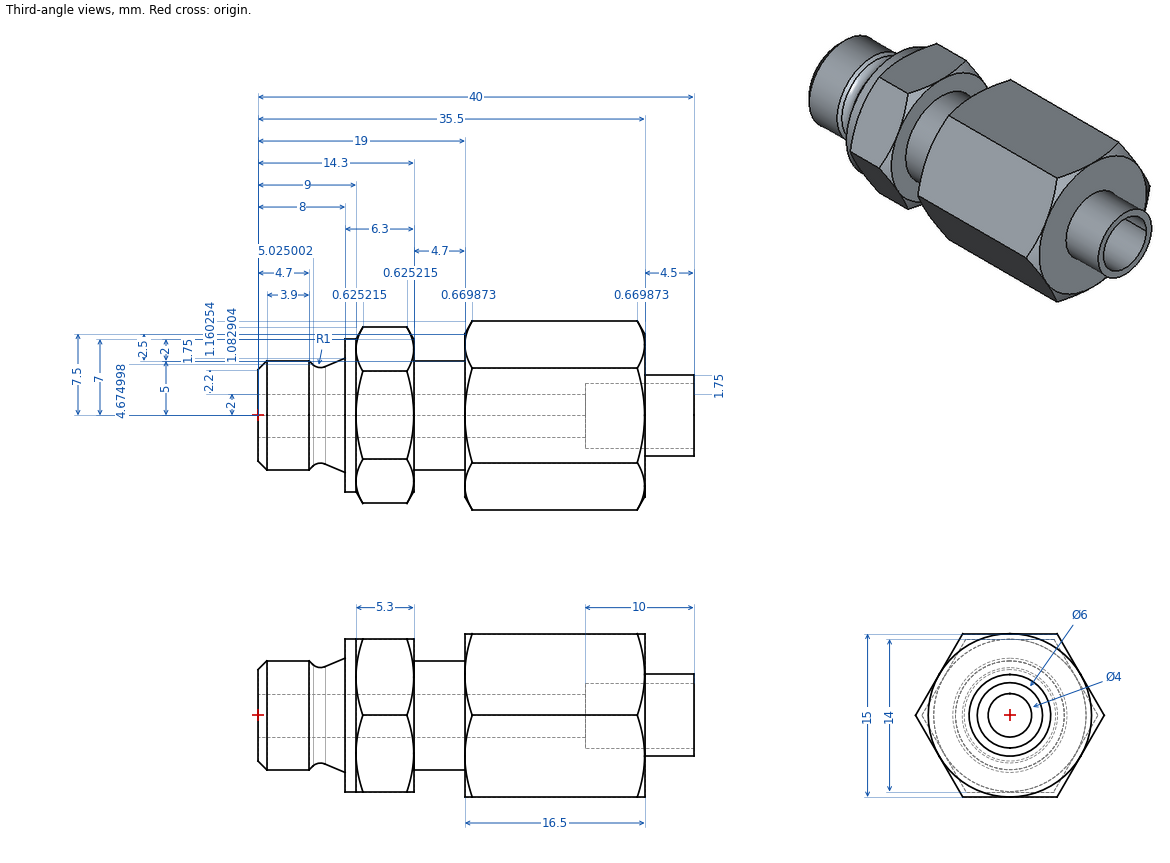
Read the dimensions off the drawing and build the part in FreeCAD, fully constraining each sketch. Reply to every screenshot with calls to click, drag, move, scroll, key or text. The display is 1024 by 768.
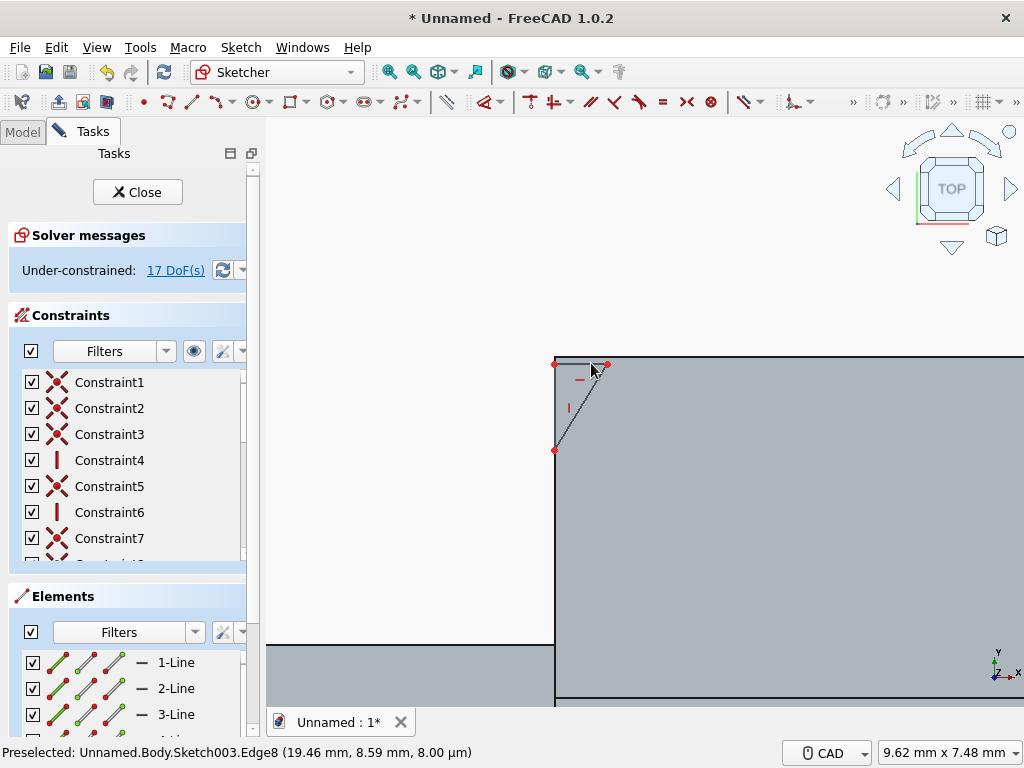
scroll(595, 367, down, 10)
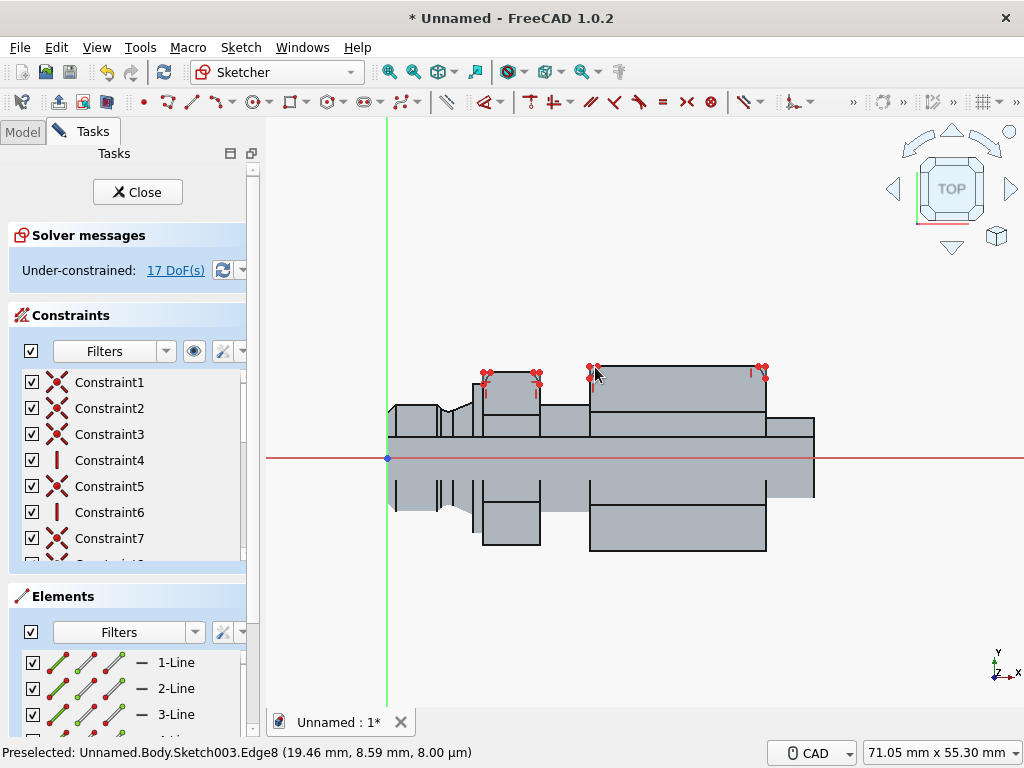
scroll(764, 366, up, 10)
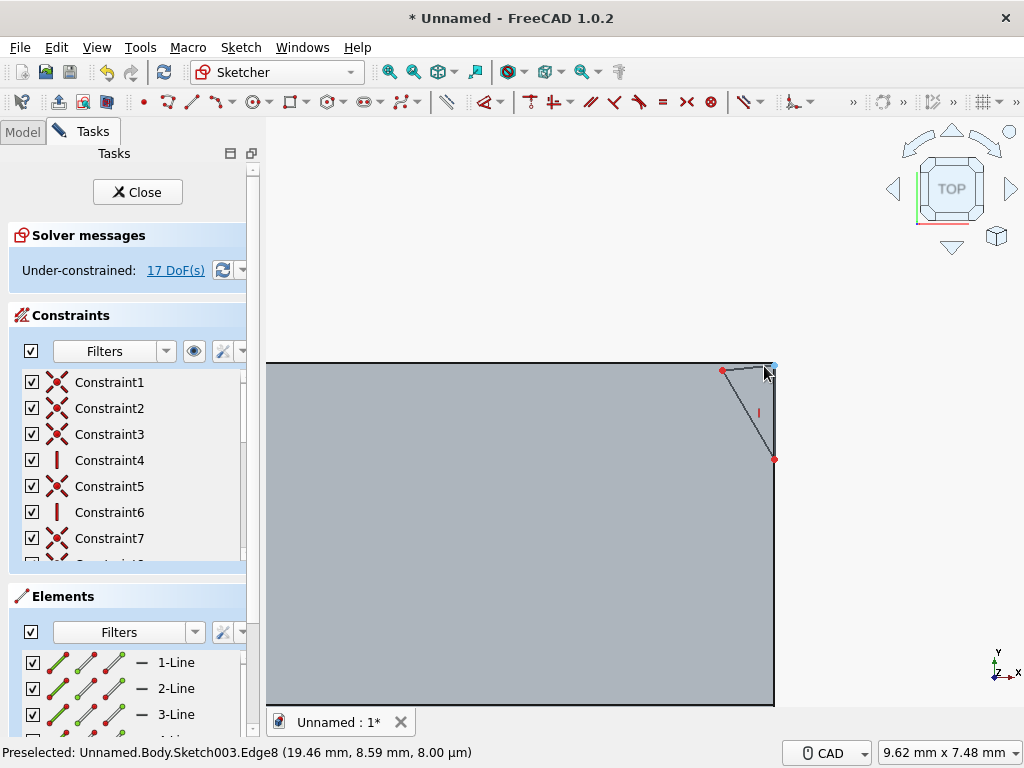
click(759, 367)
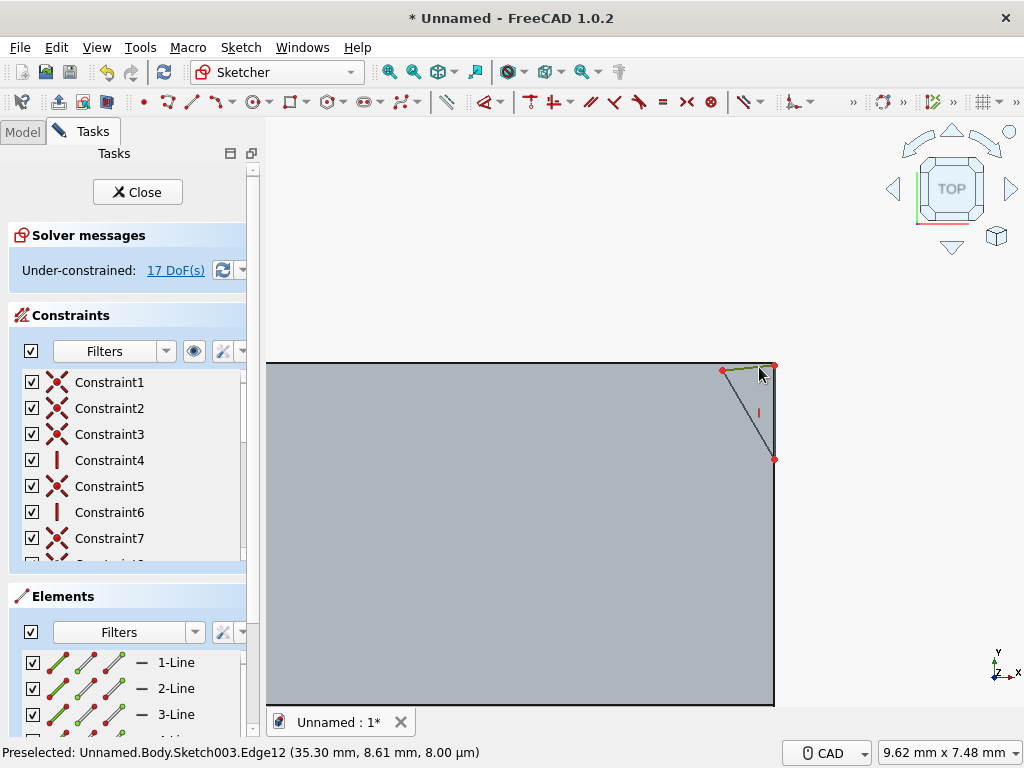
key(h)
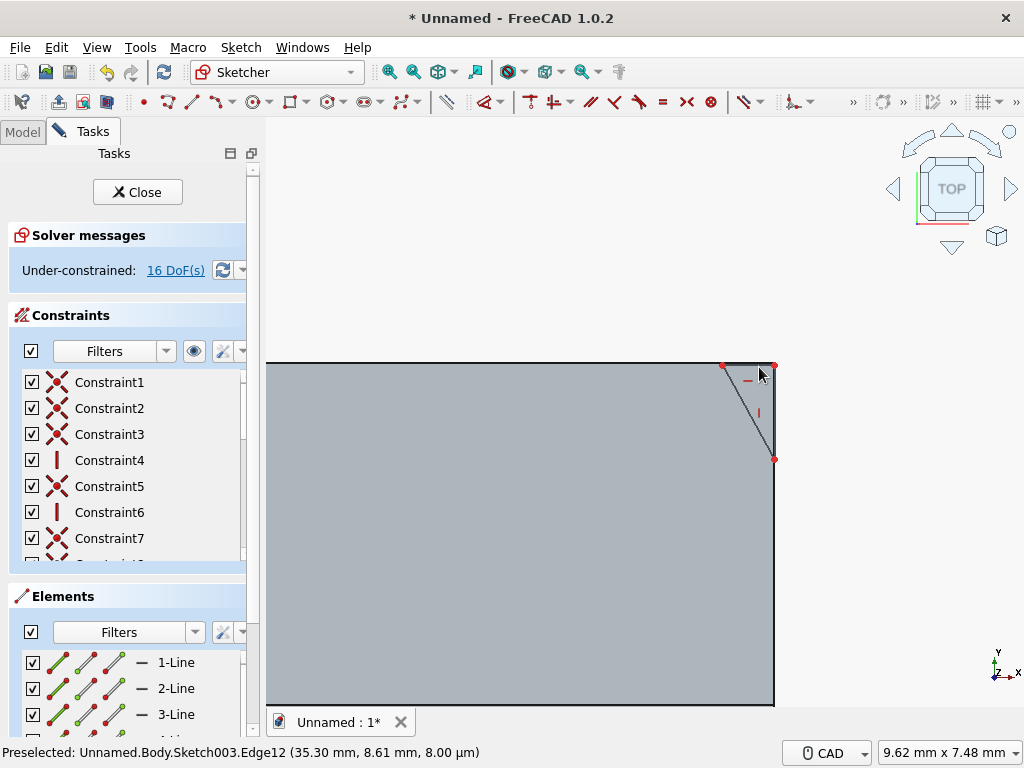
key(d)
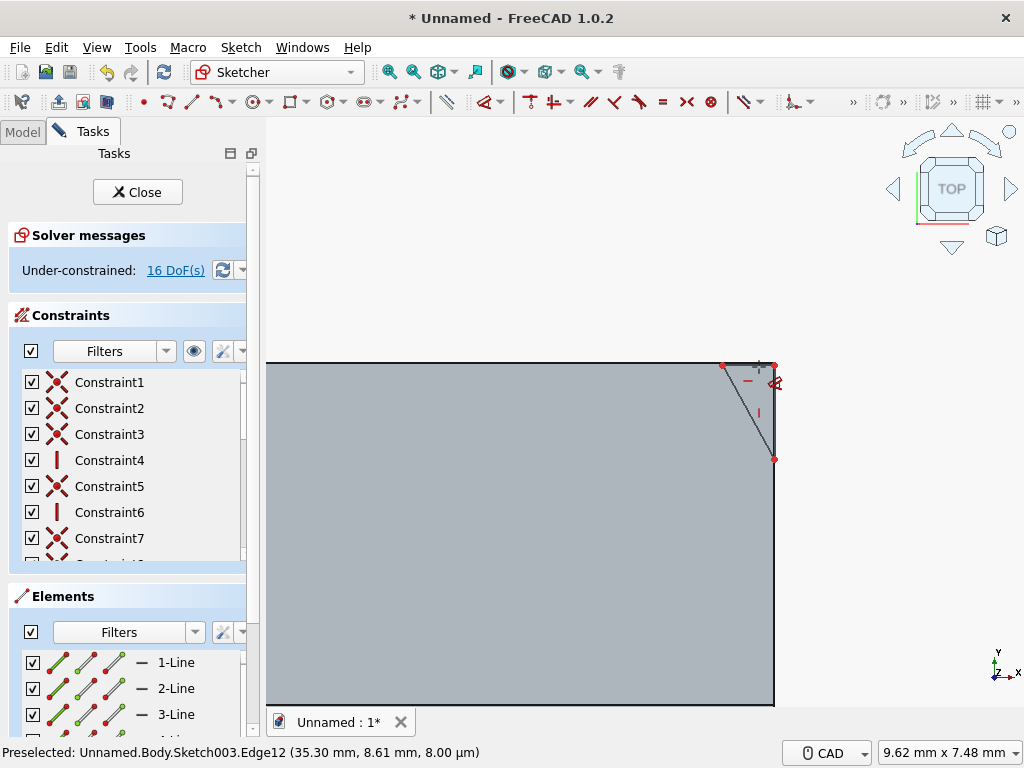
scroll(765, 366, down, 10)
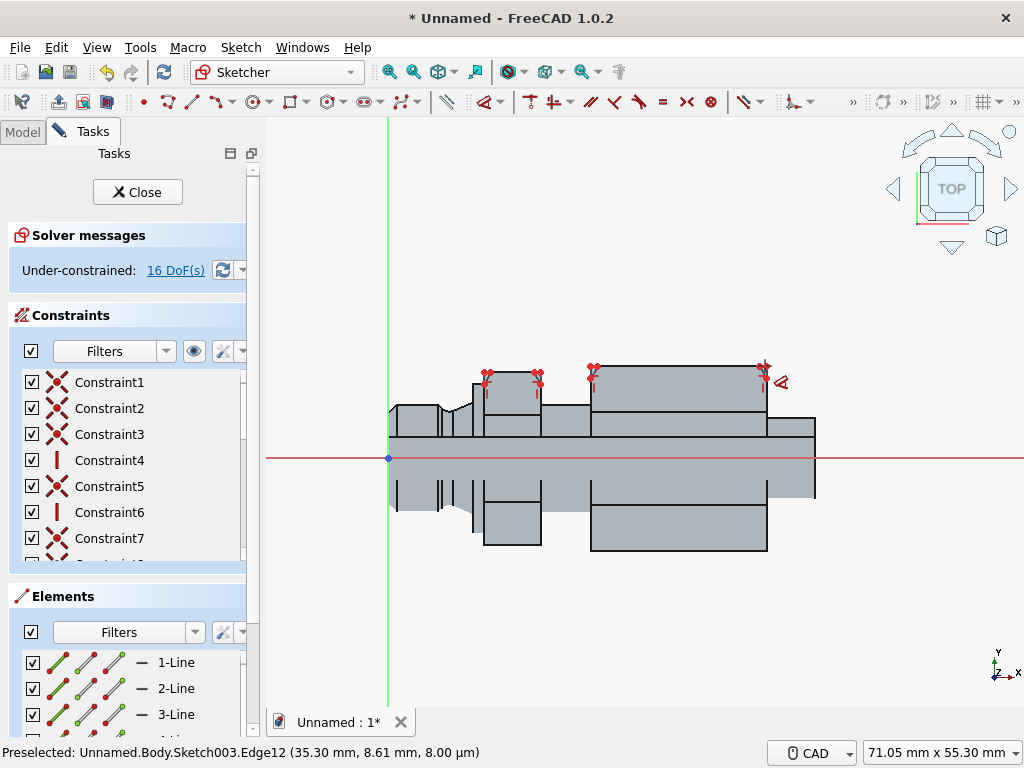
click(484, 385)
click(436, 492)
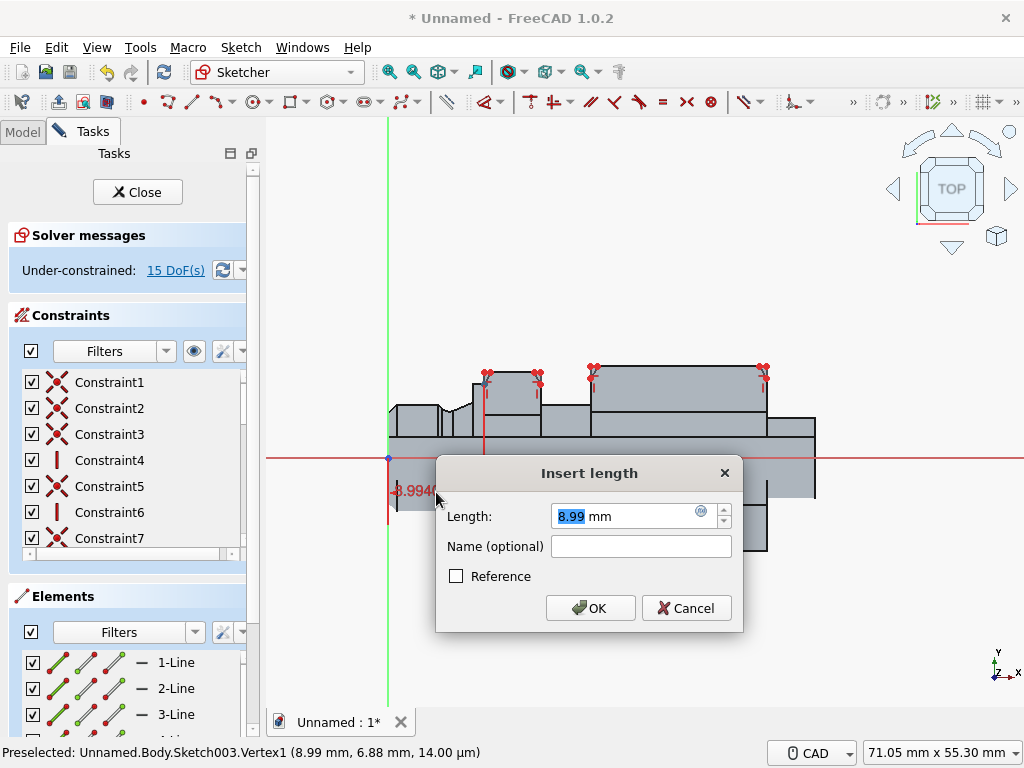
text(9)
key(Return)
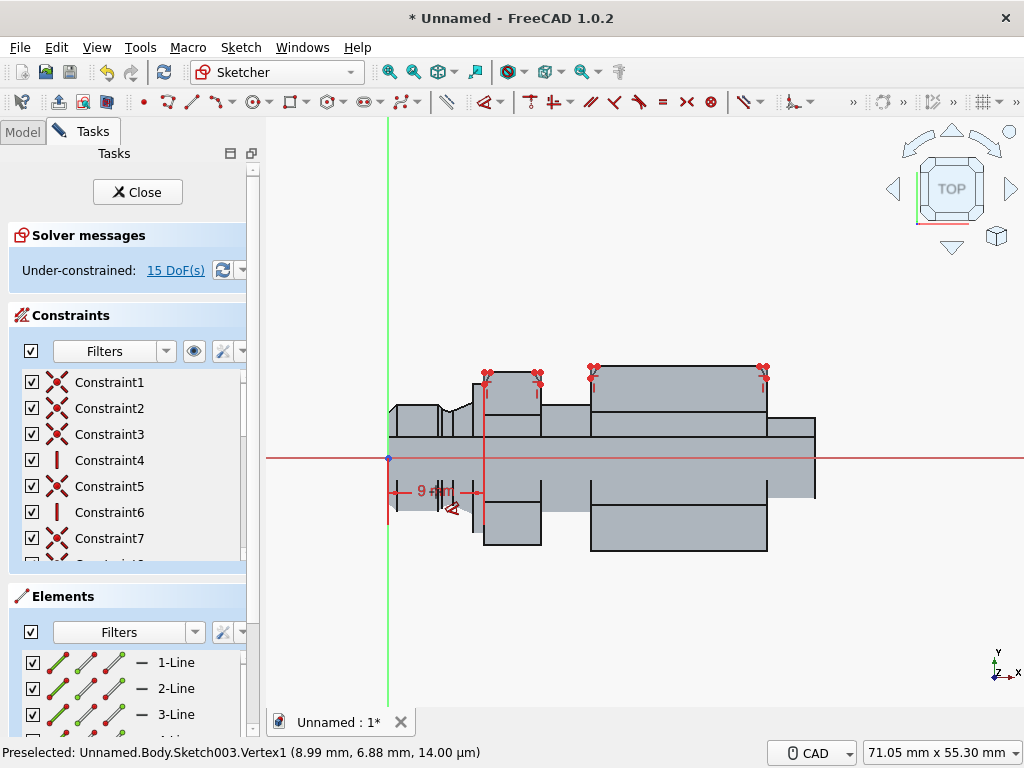
click(484, 385)
click(354, 422)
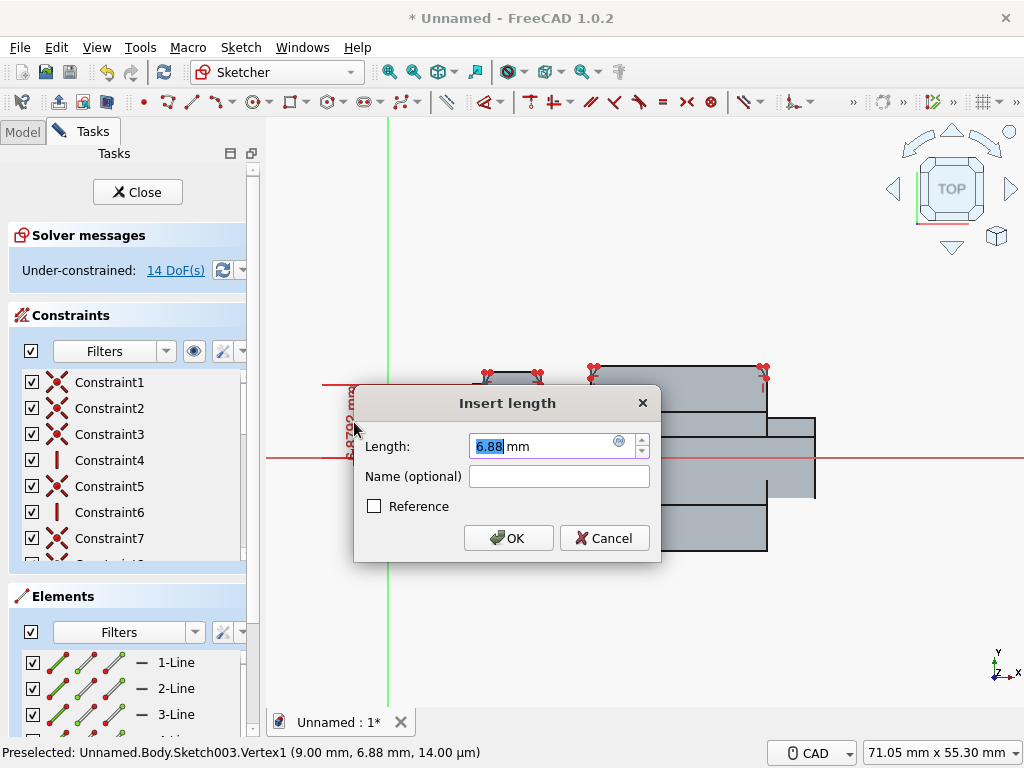
text(7)
key(Return)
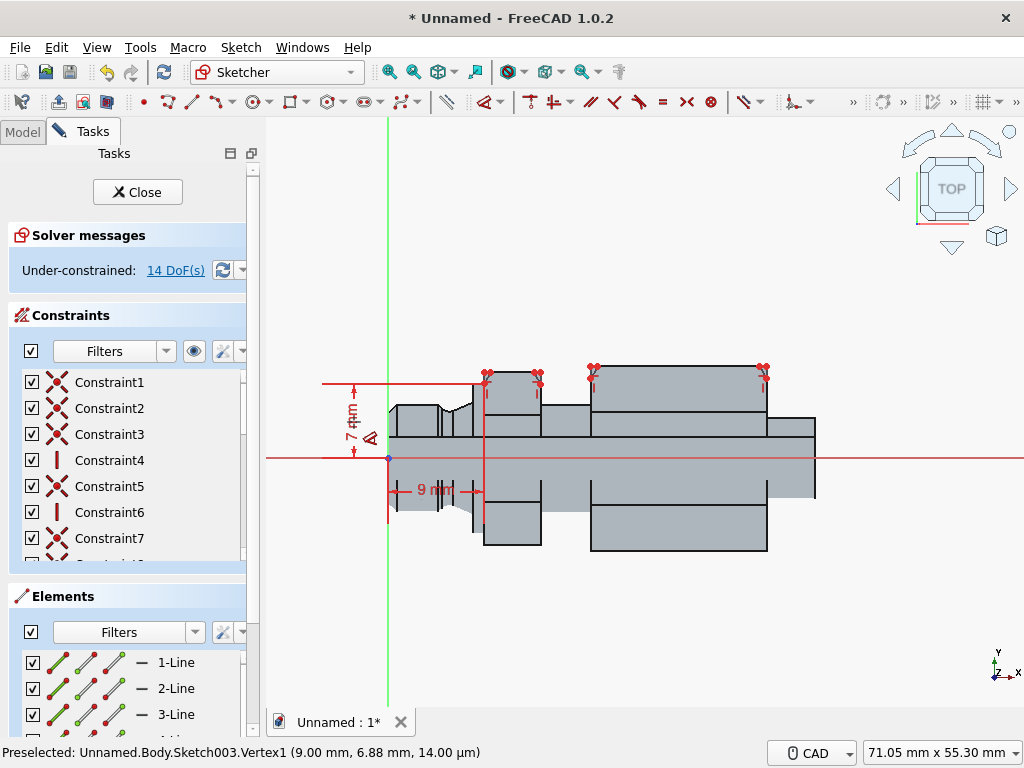
click(541, 384)
click(354, 395)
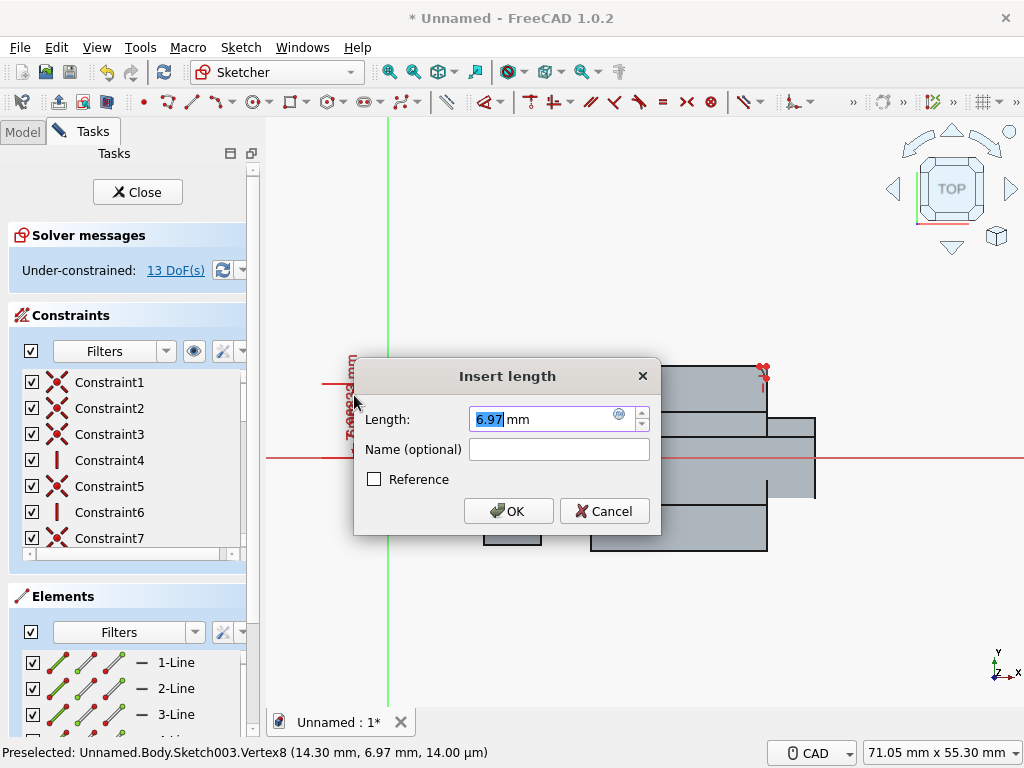
text(7)
key(Return)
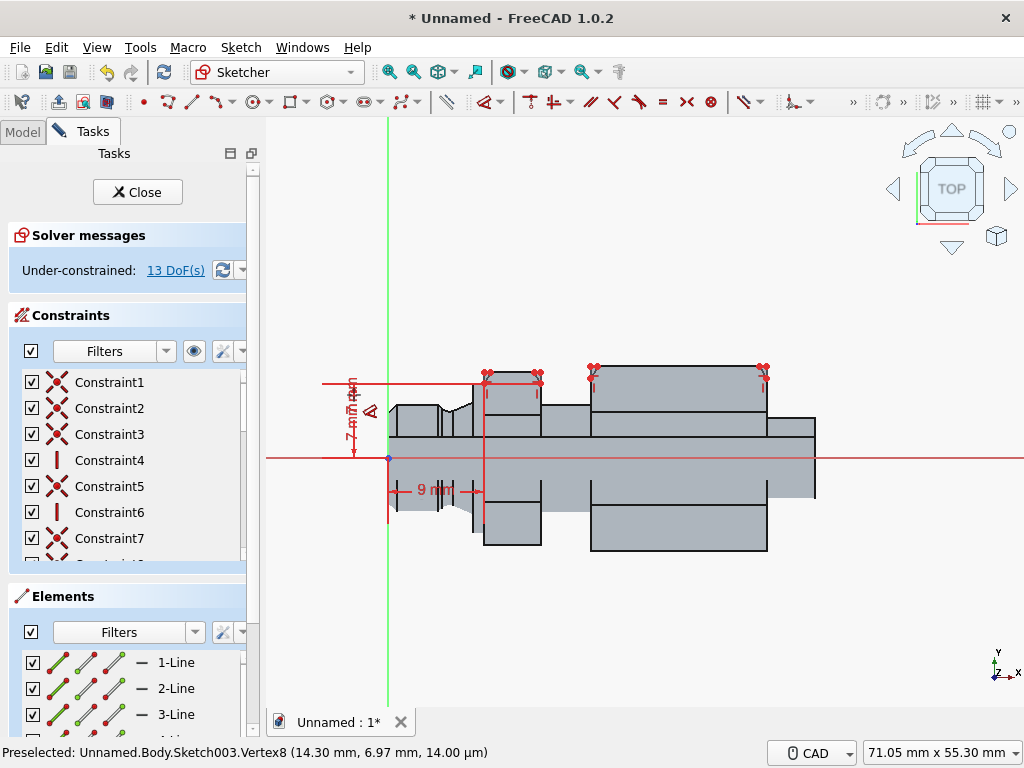
click(591, 379)
click(536, 492)